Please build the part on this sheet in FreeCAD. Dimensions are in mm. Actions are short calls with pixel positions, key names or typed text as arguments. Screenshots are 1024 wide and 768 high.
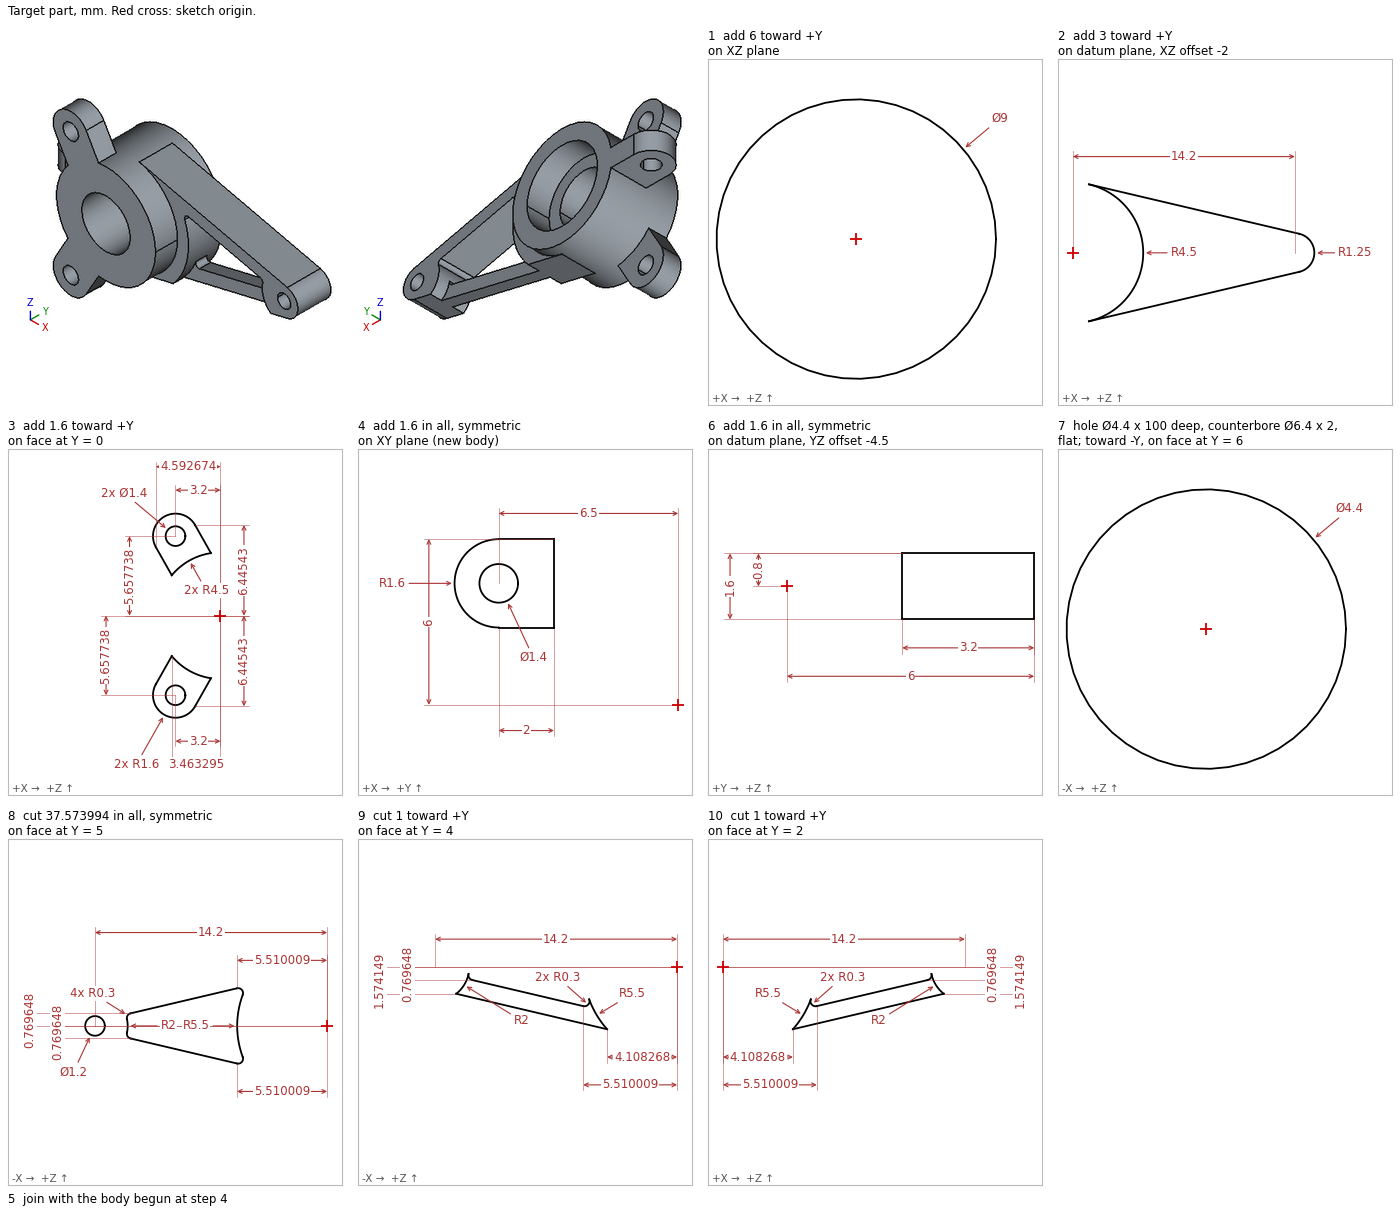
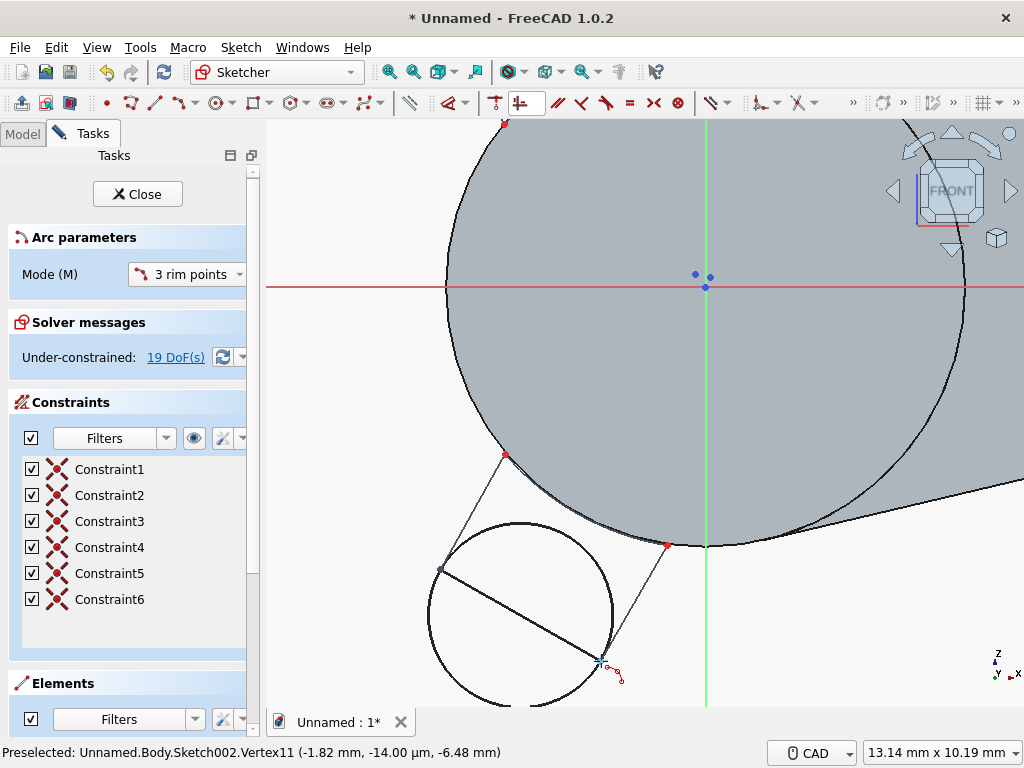
scroll(579, 516, down, 4)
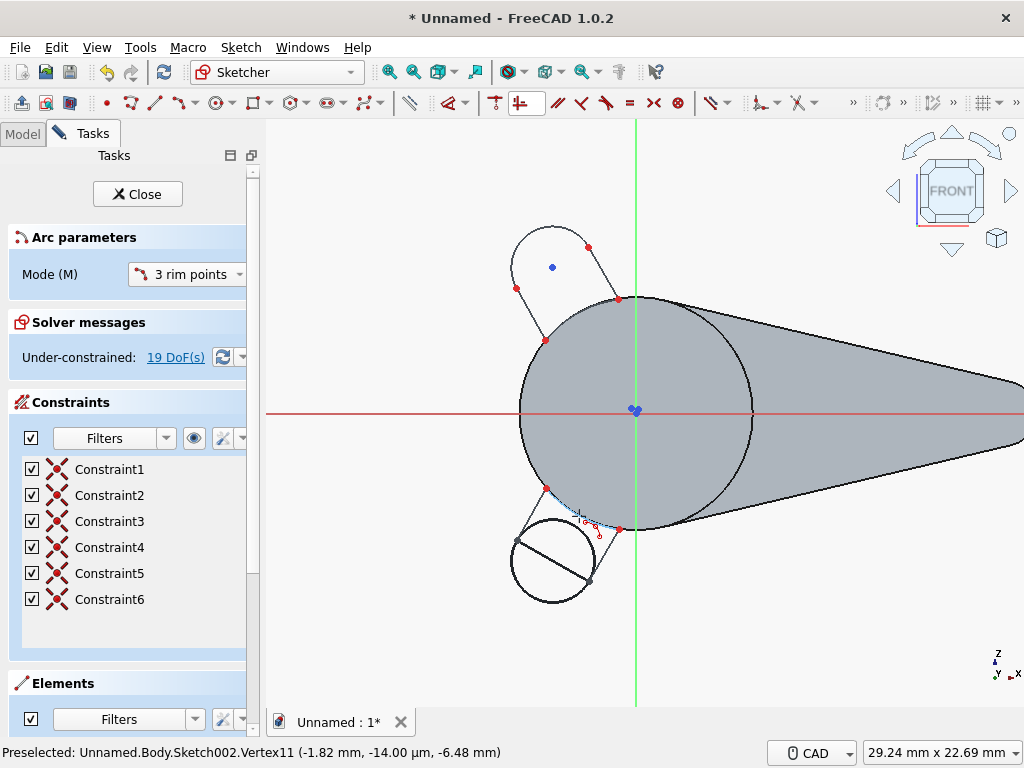
click(533, 596)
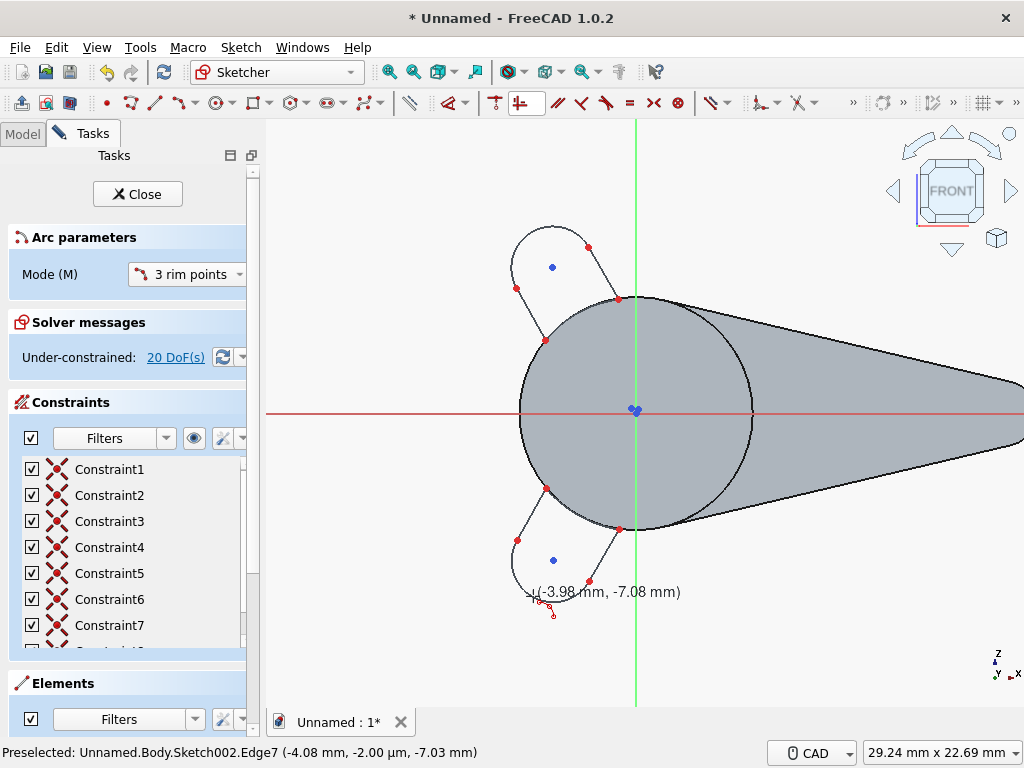
key(g)
key(c)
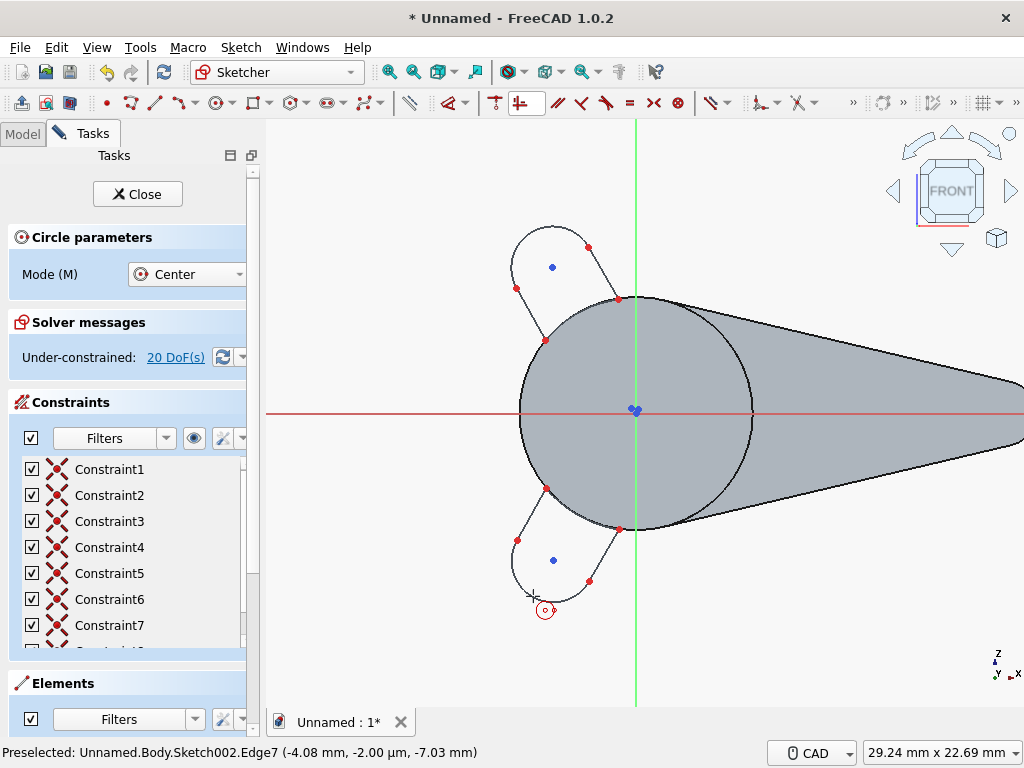
scroll(553, 267, up, 2)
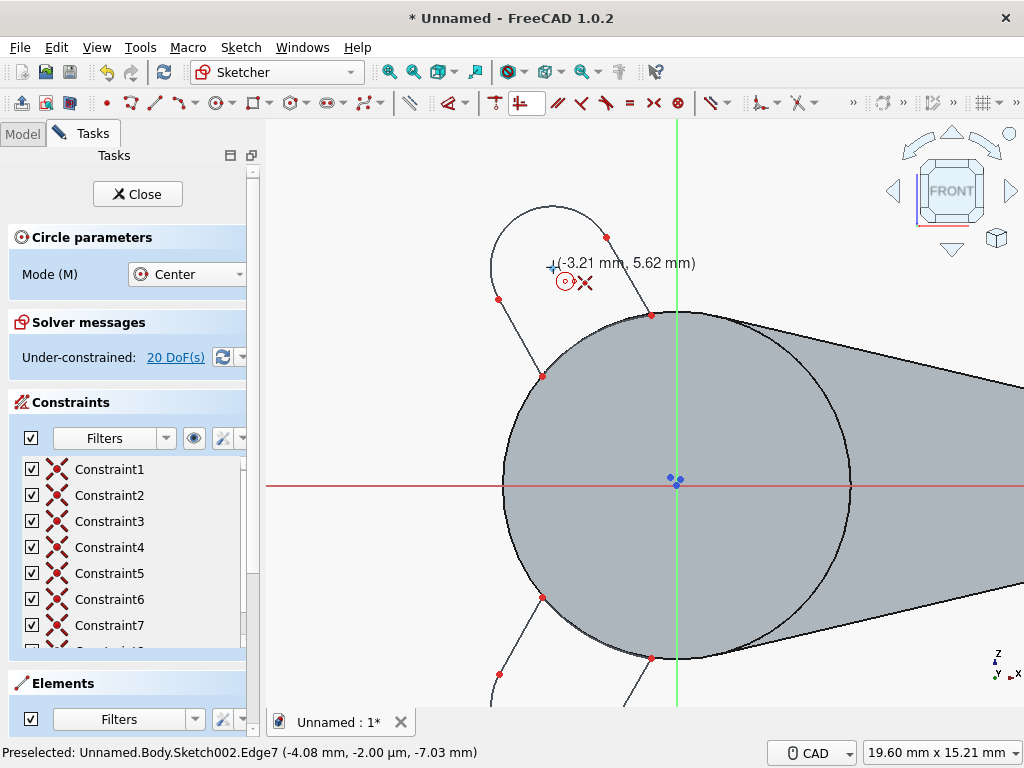
click(553, 267)
click(572, 248)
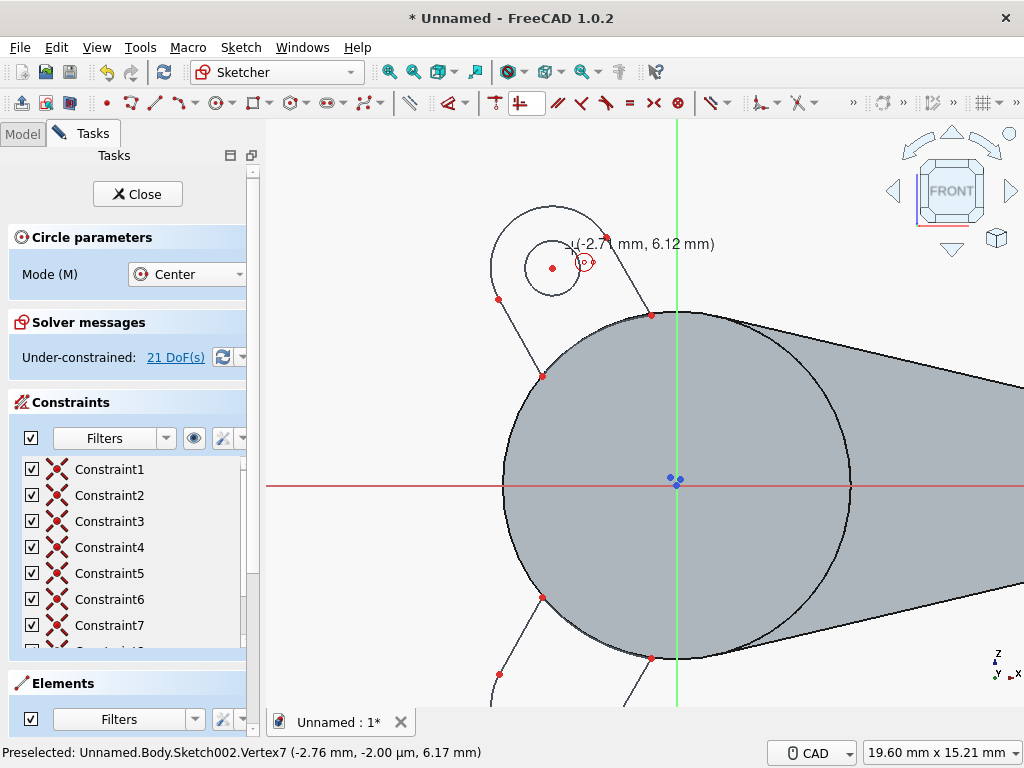
scroll(553, 266, down, 2)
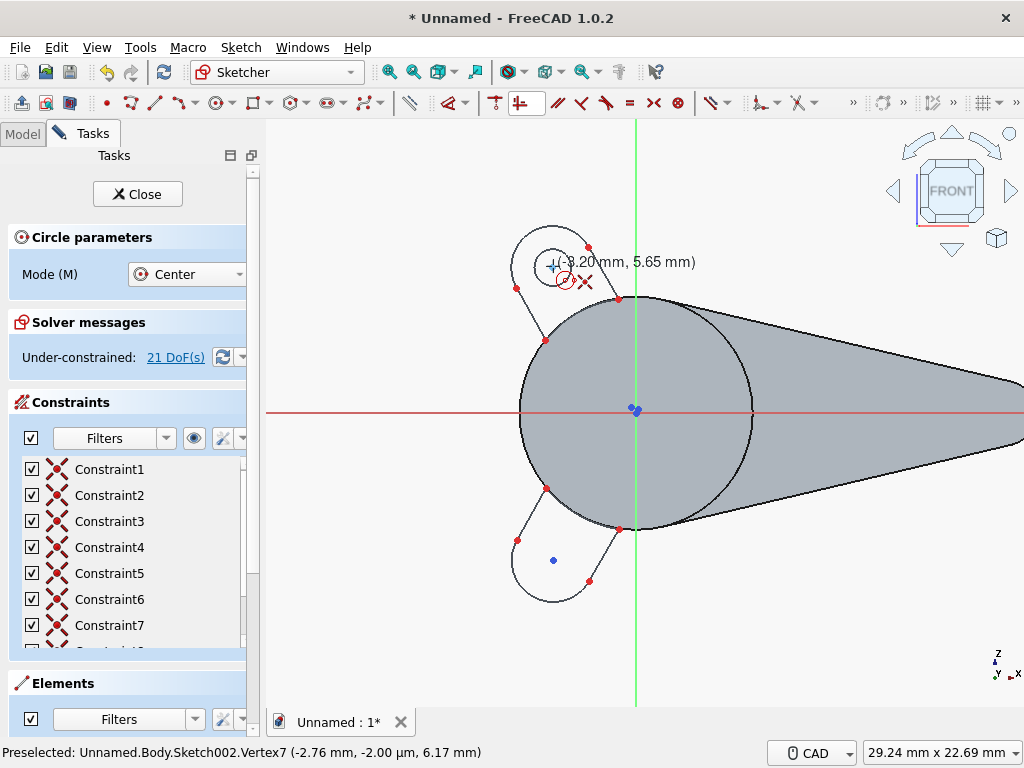
scroll(553, 560, up, 2)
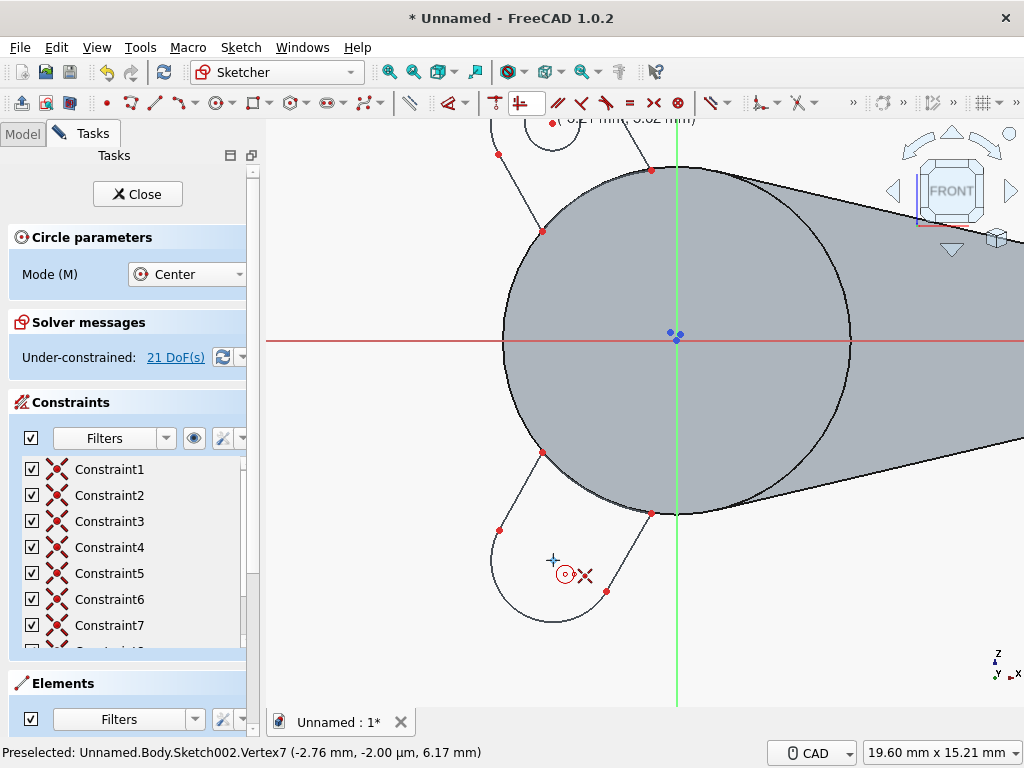
click(553, 559)
click(572, 540)
key(Escape)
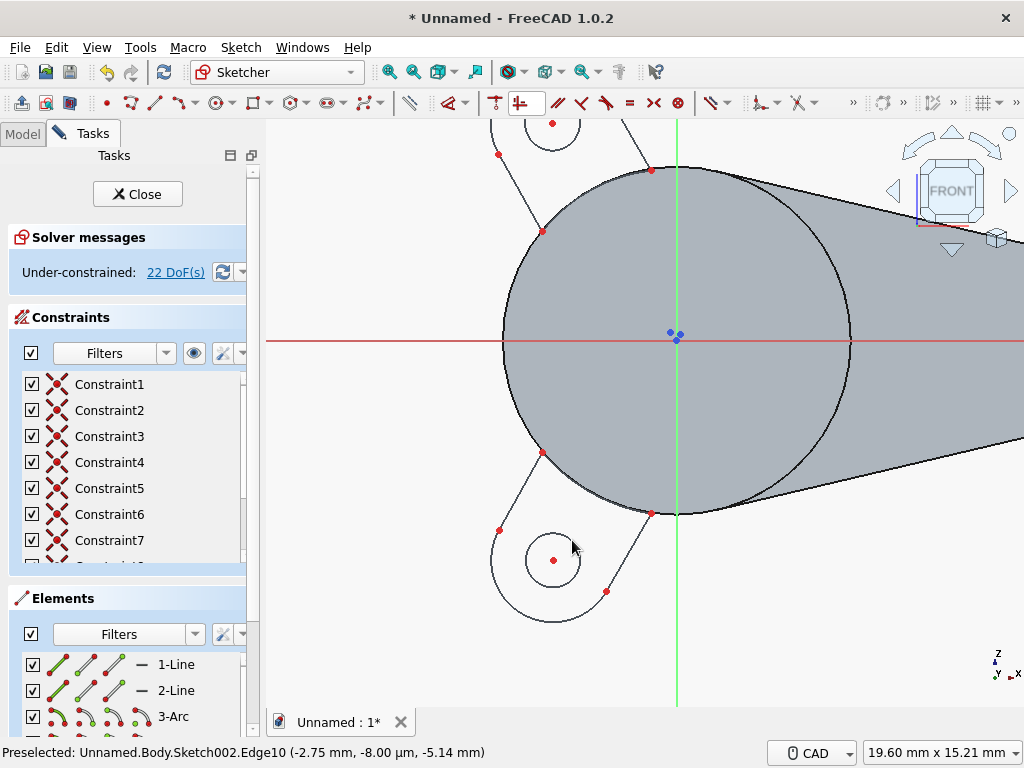
click(638, 147)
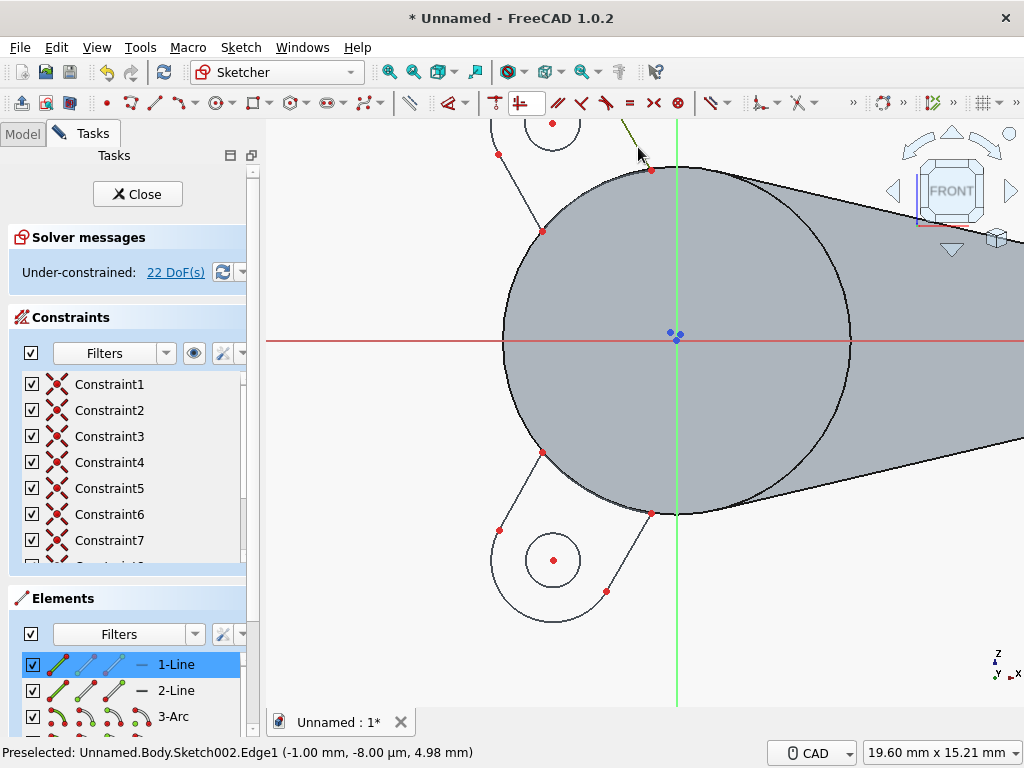
scroll(553, 560, down, 2)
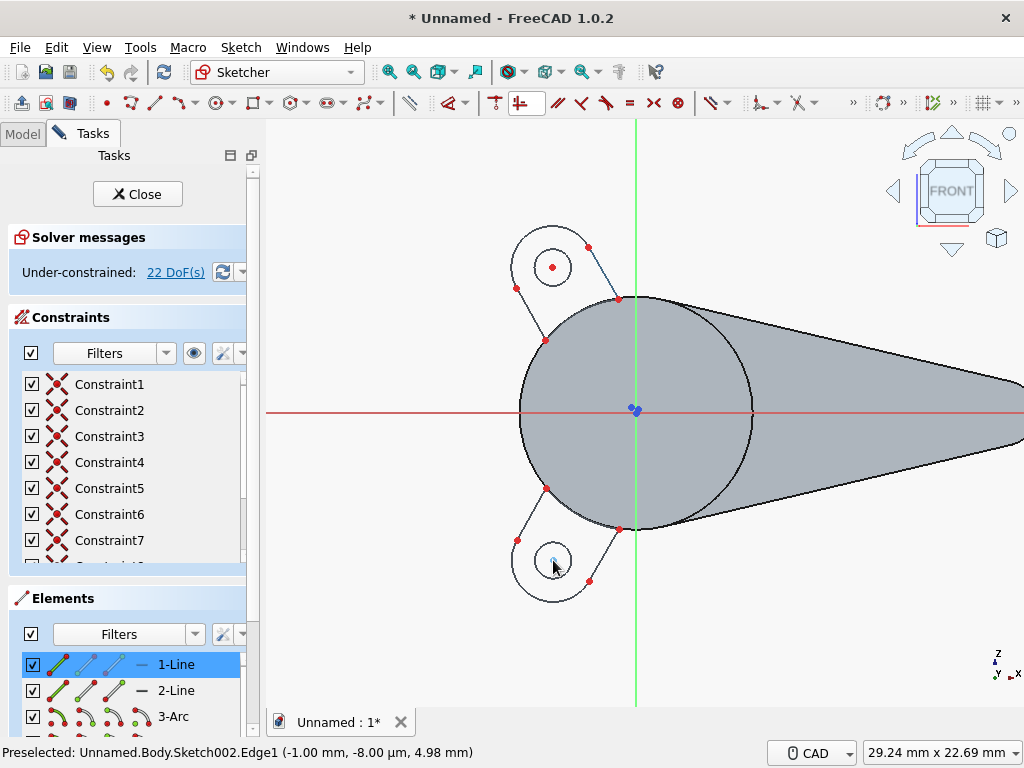
click(557, 226)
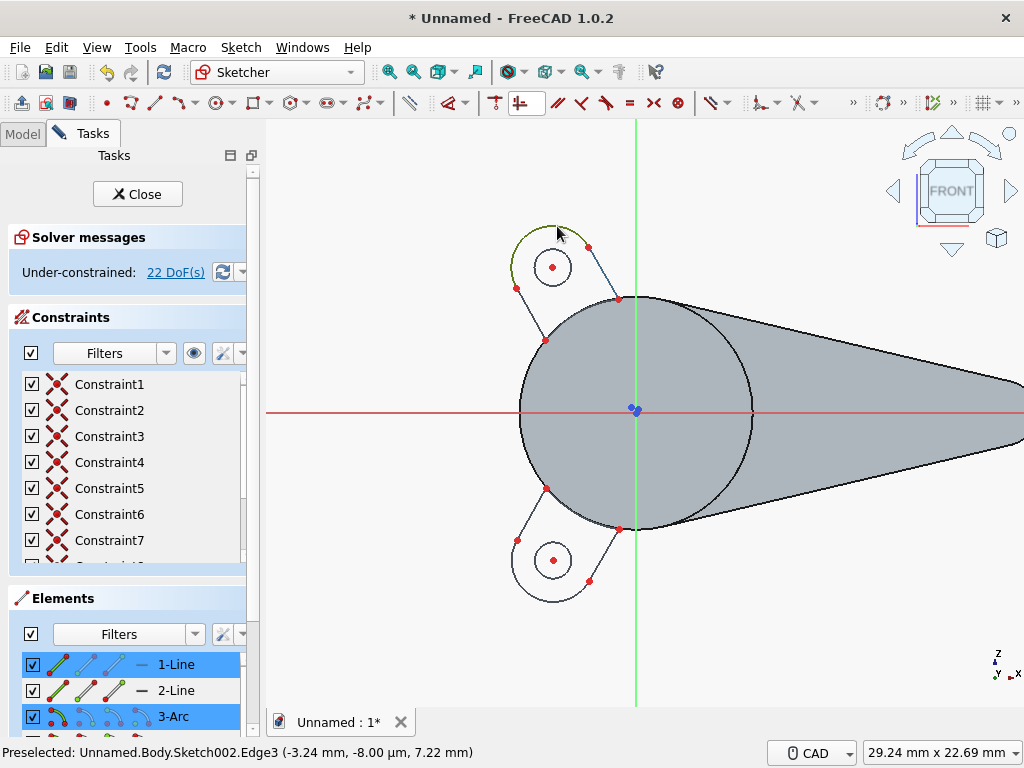
click(606, 104)